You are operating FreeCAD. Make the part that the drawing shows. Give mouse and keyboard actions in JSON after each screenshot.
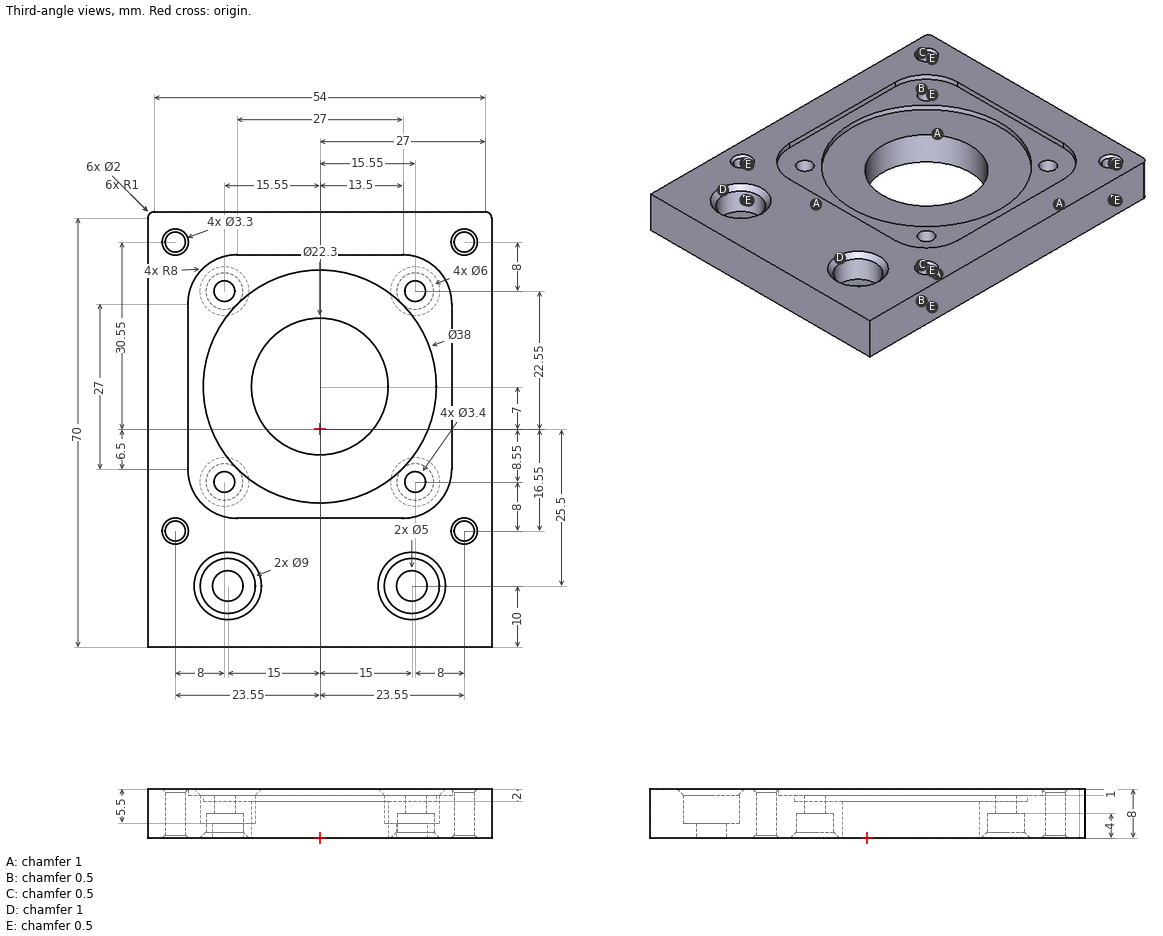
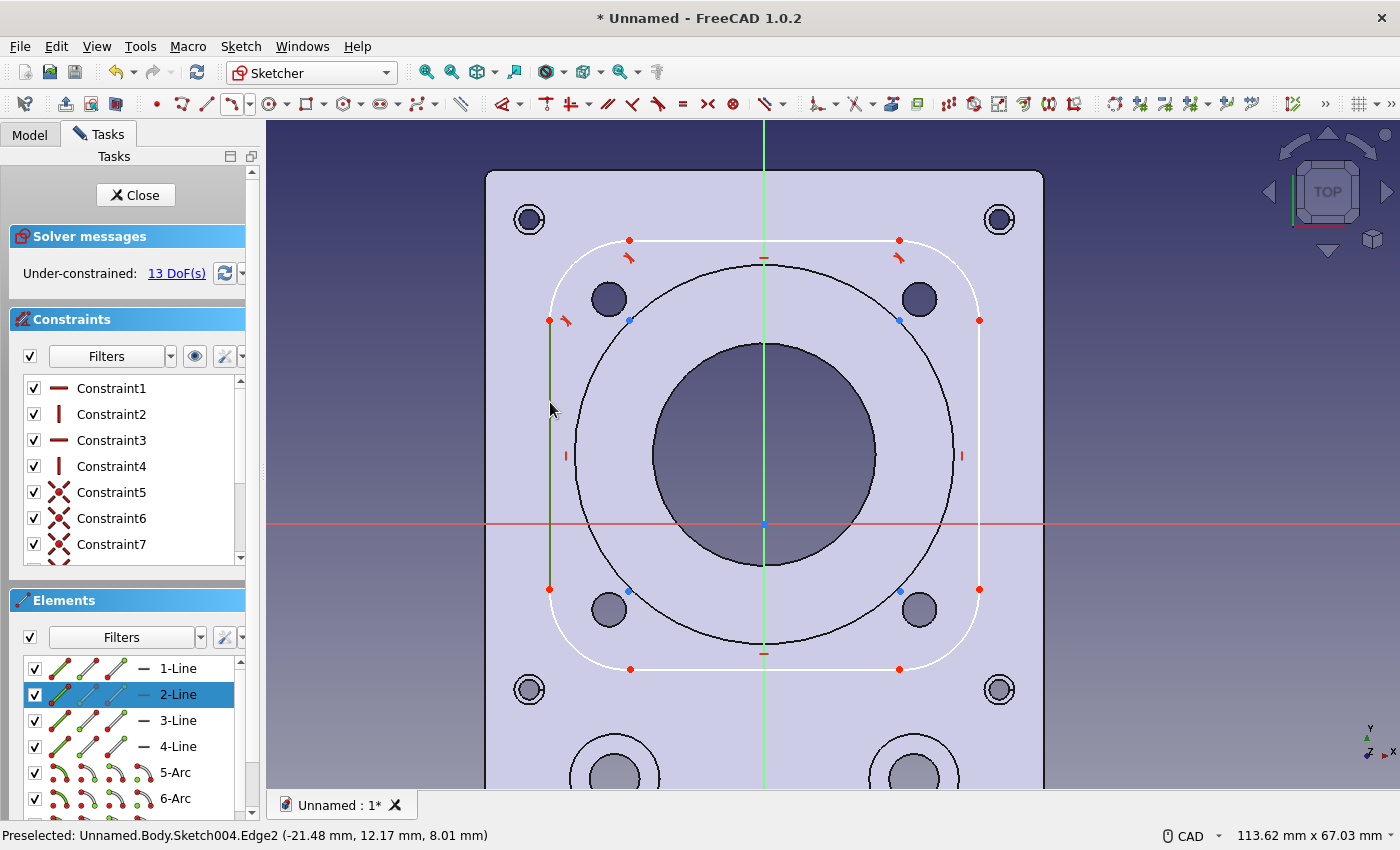
{"action": "left_click", "coordinate": [558, 627]}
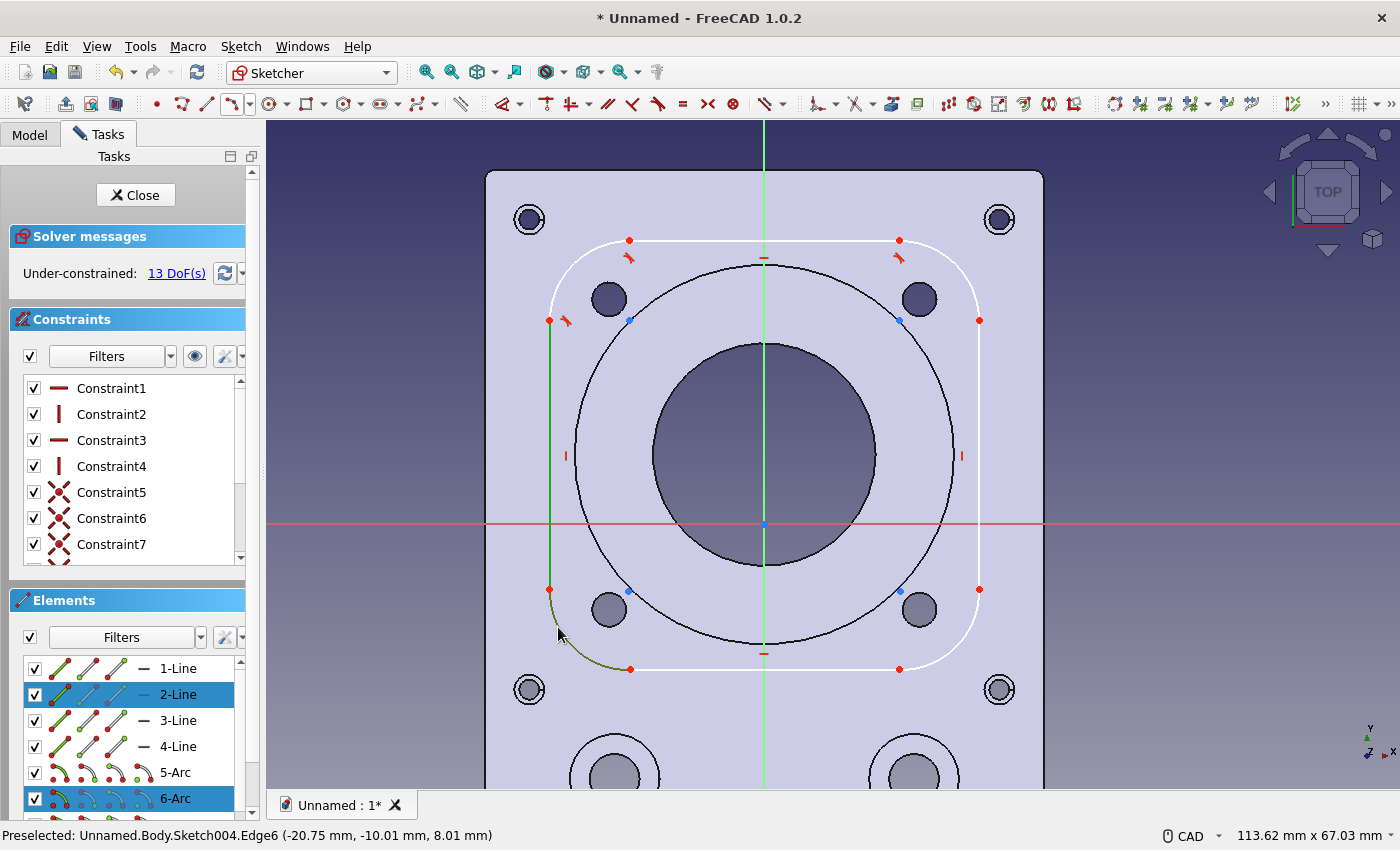
{"action": "key", "text": "t"}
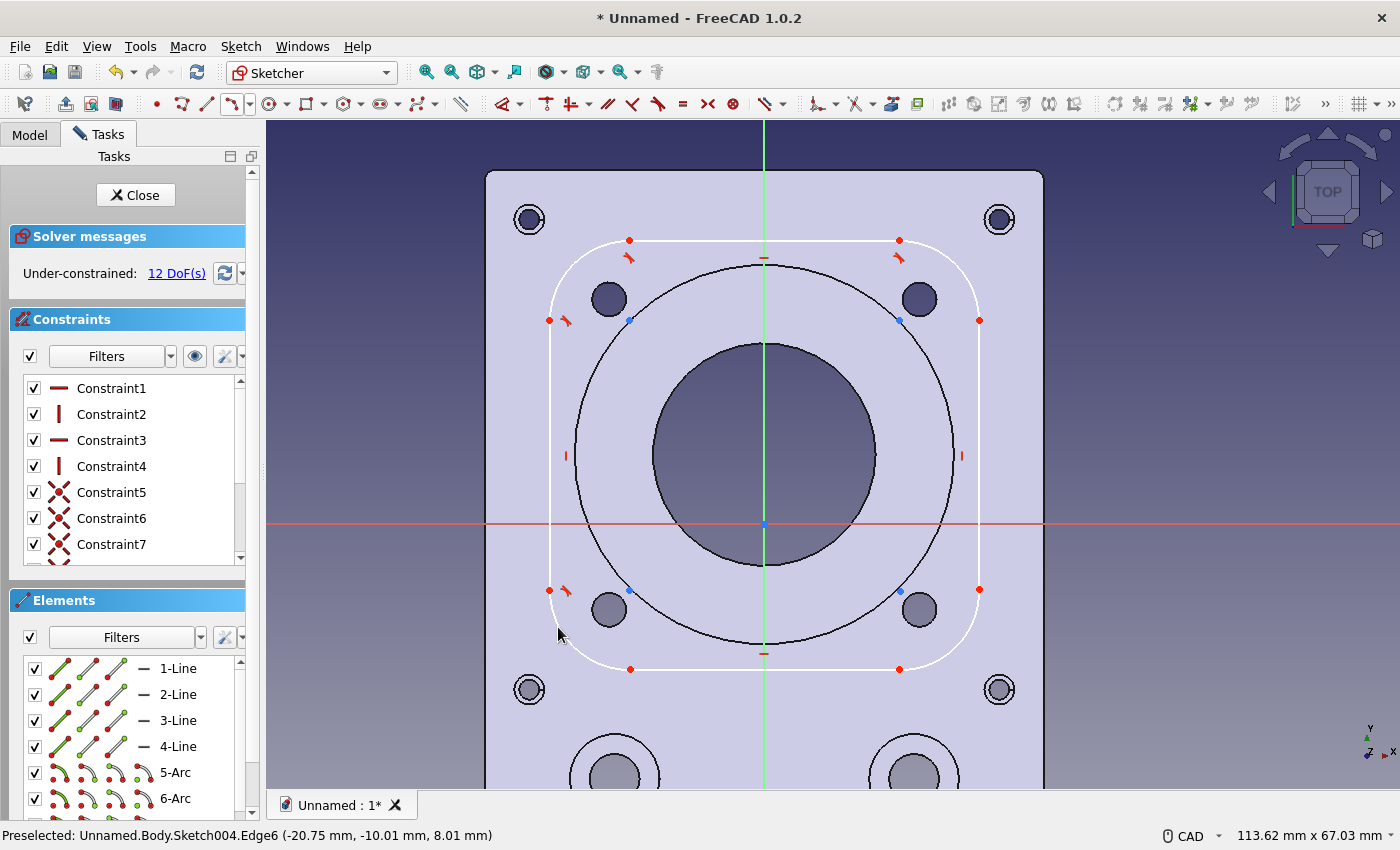
{"action": "left_click", "coordinate": [711, 670]}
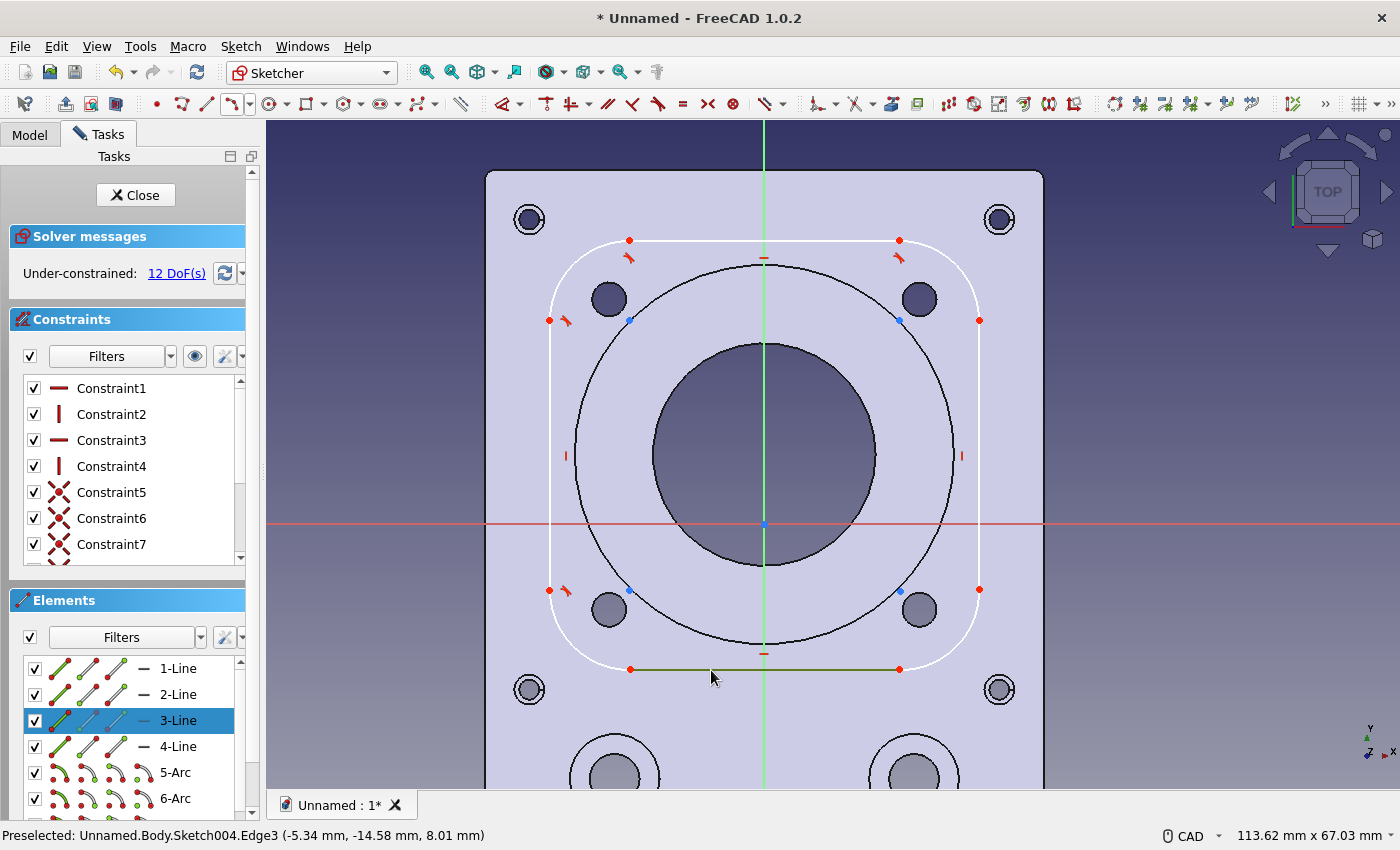
{"action": "left_click", "coordinate": [559, 626]}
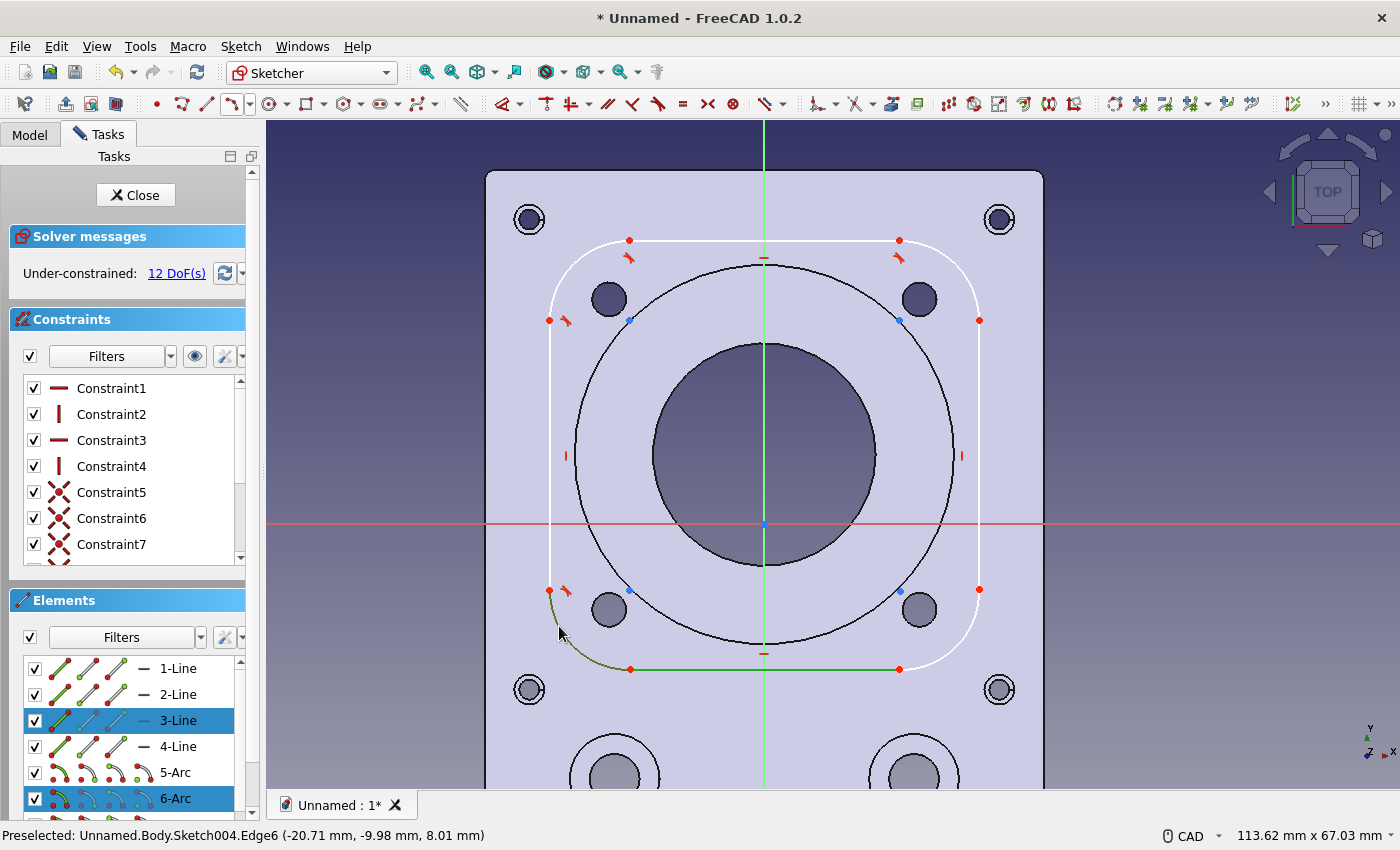
{"action": "key", "text": "t"}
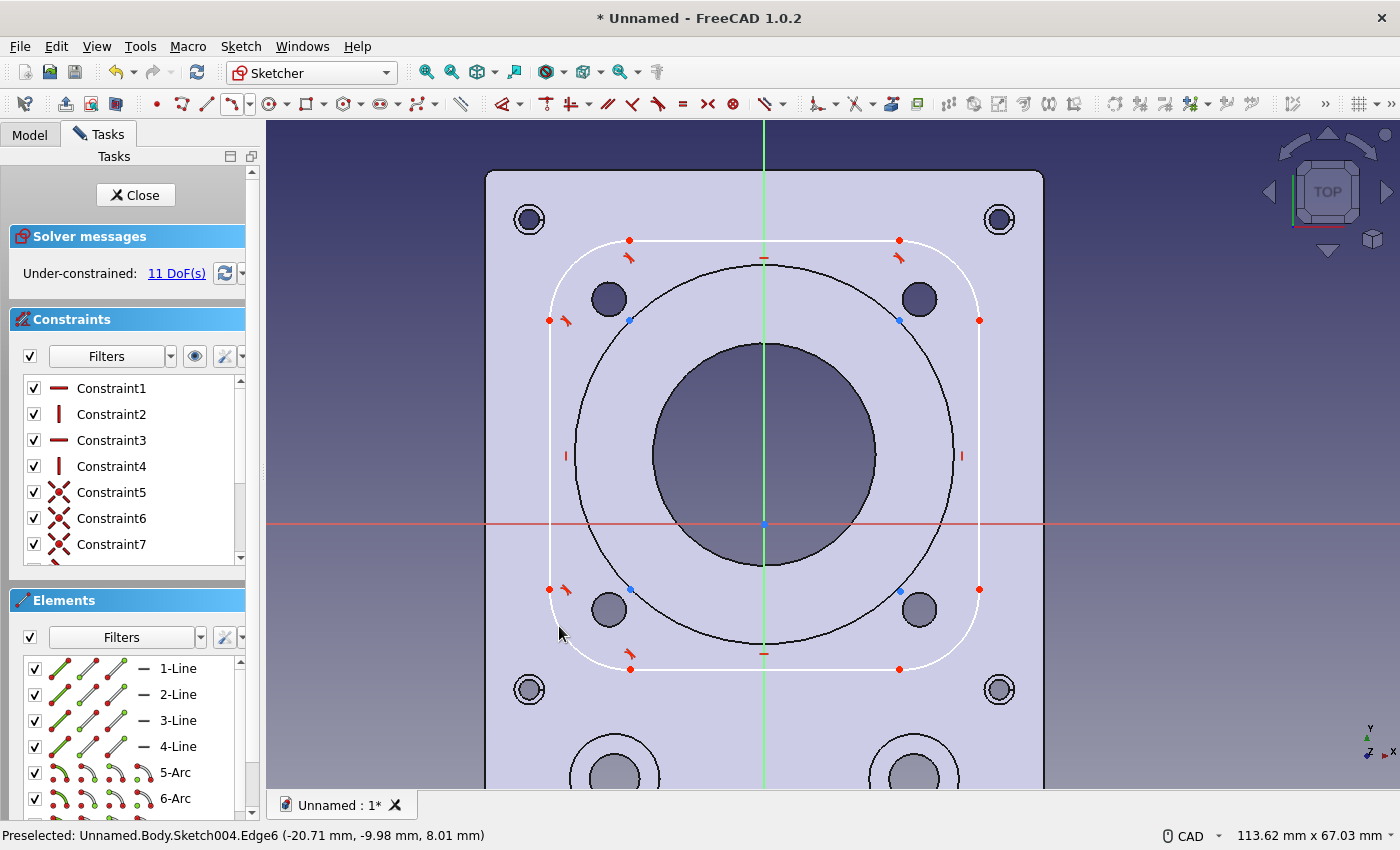
{"action": "left_click", "coordinate": [711, 670]}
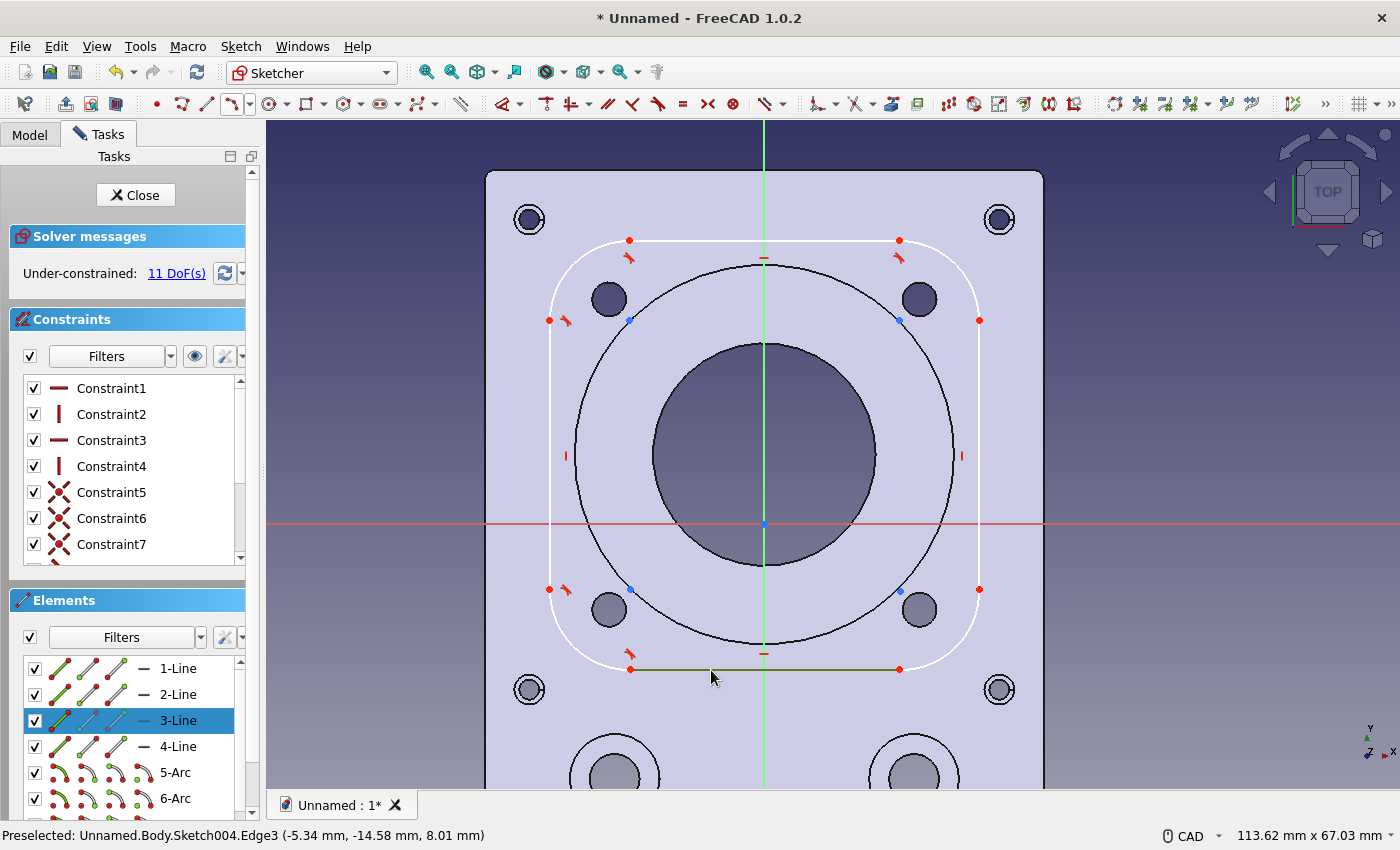
{"action": "left_click", "coordinate": [936, 662]}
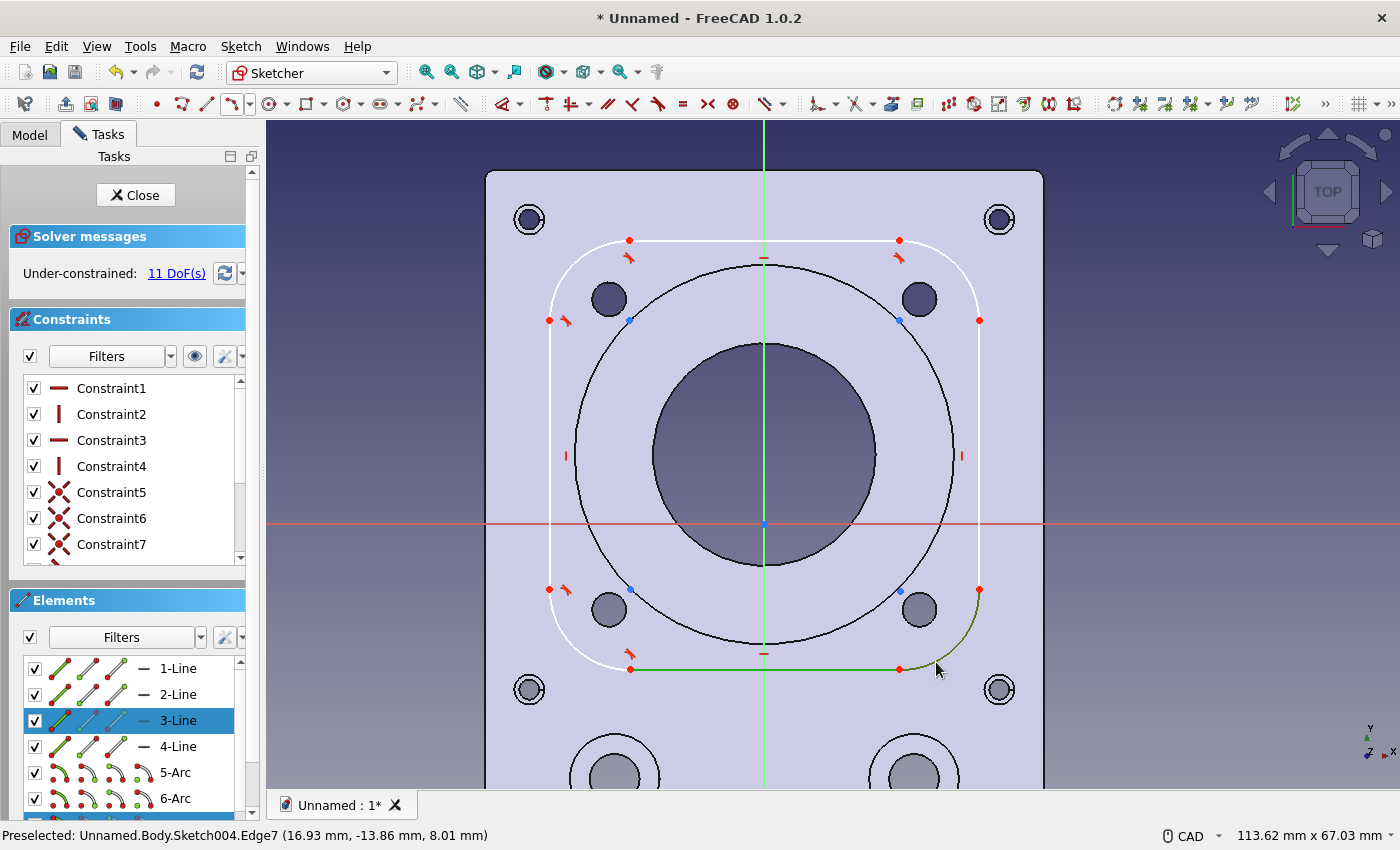
{"action": "left_click", "coordinate": [658, 104]}